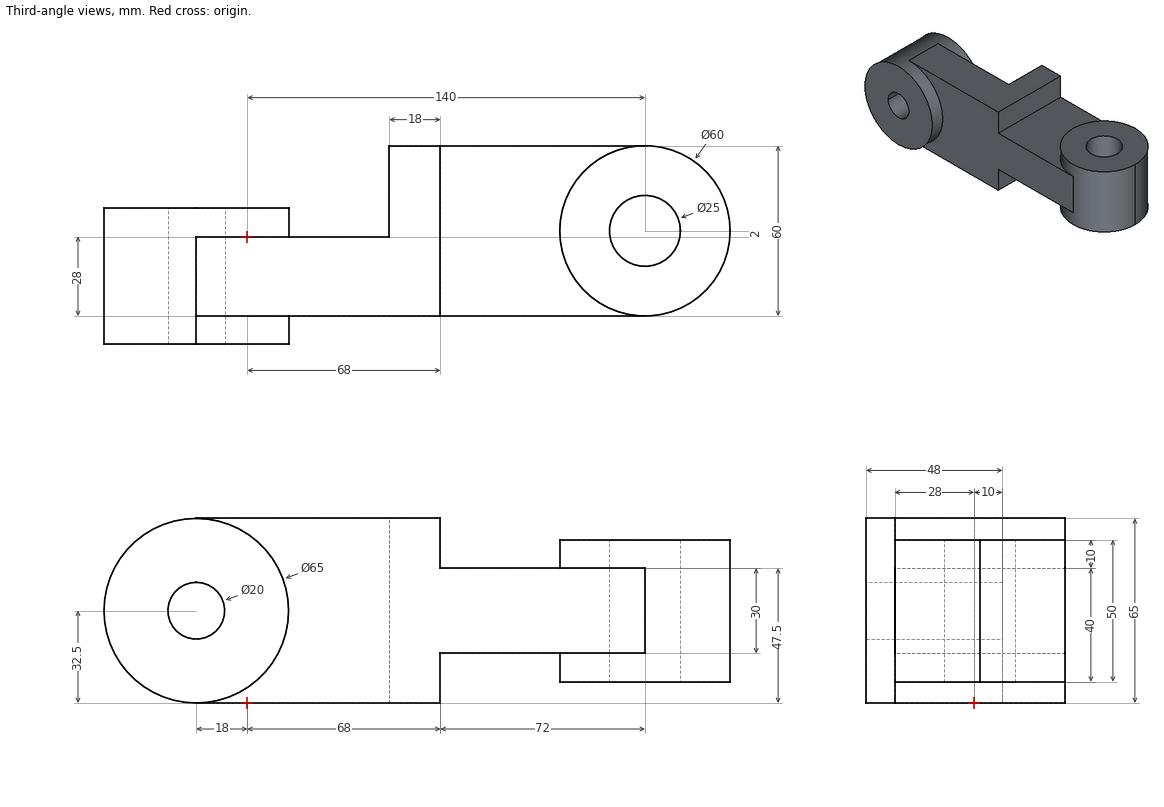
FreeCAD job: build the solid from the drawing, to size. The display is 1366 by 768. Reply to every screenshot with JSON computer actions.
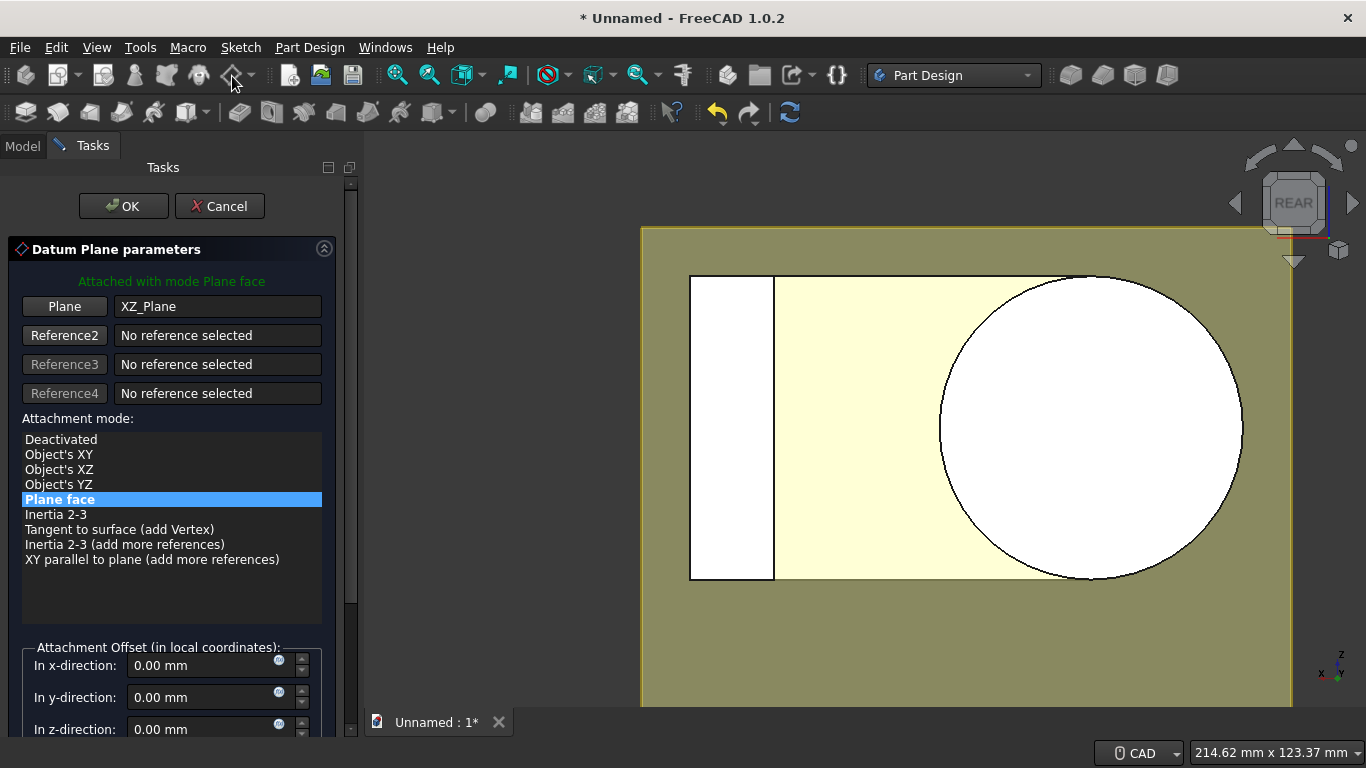
{"action": "scroll", "coordinate": [351, 456], "scroll_direction": "down", "scroll_amount": 2}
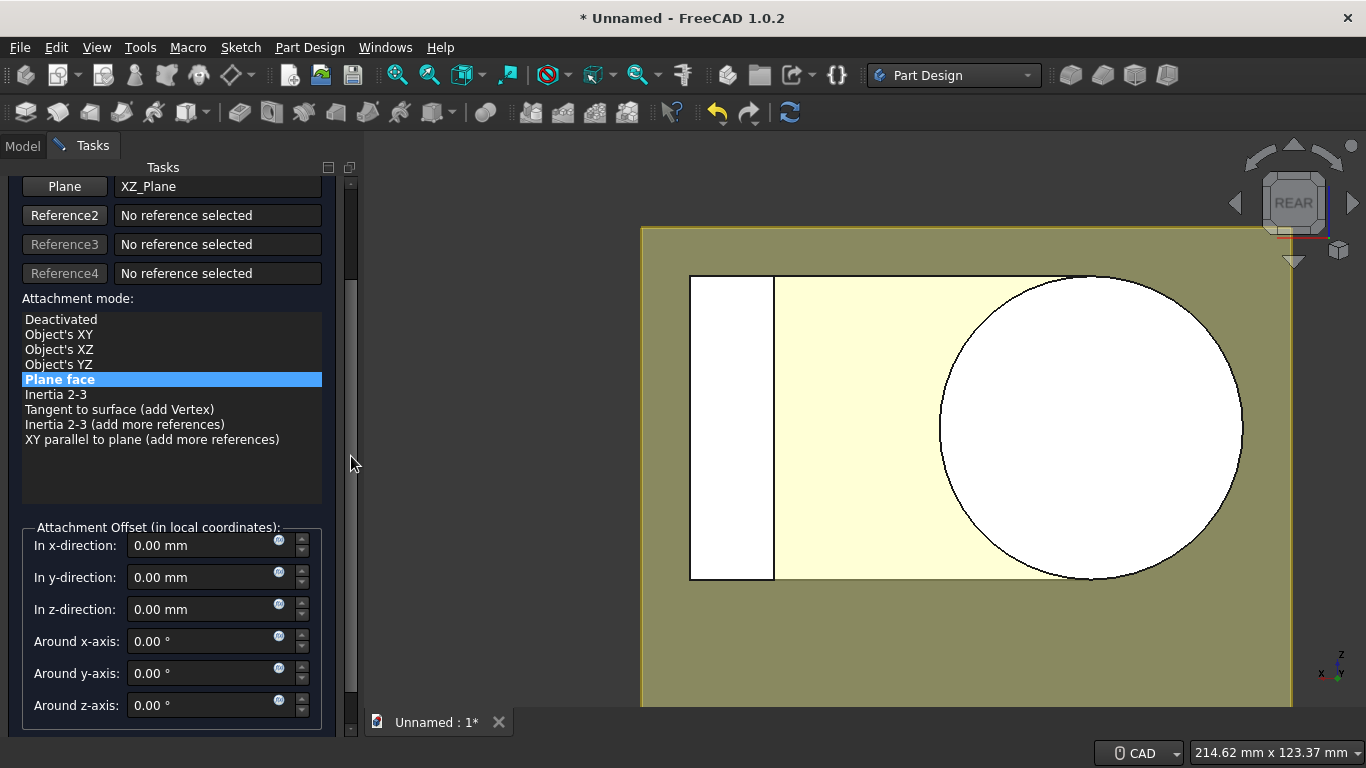
{"action": "triple_click", "coordinate": [210, 609]}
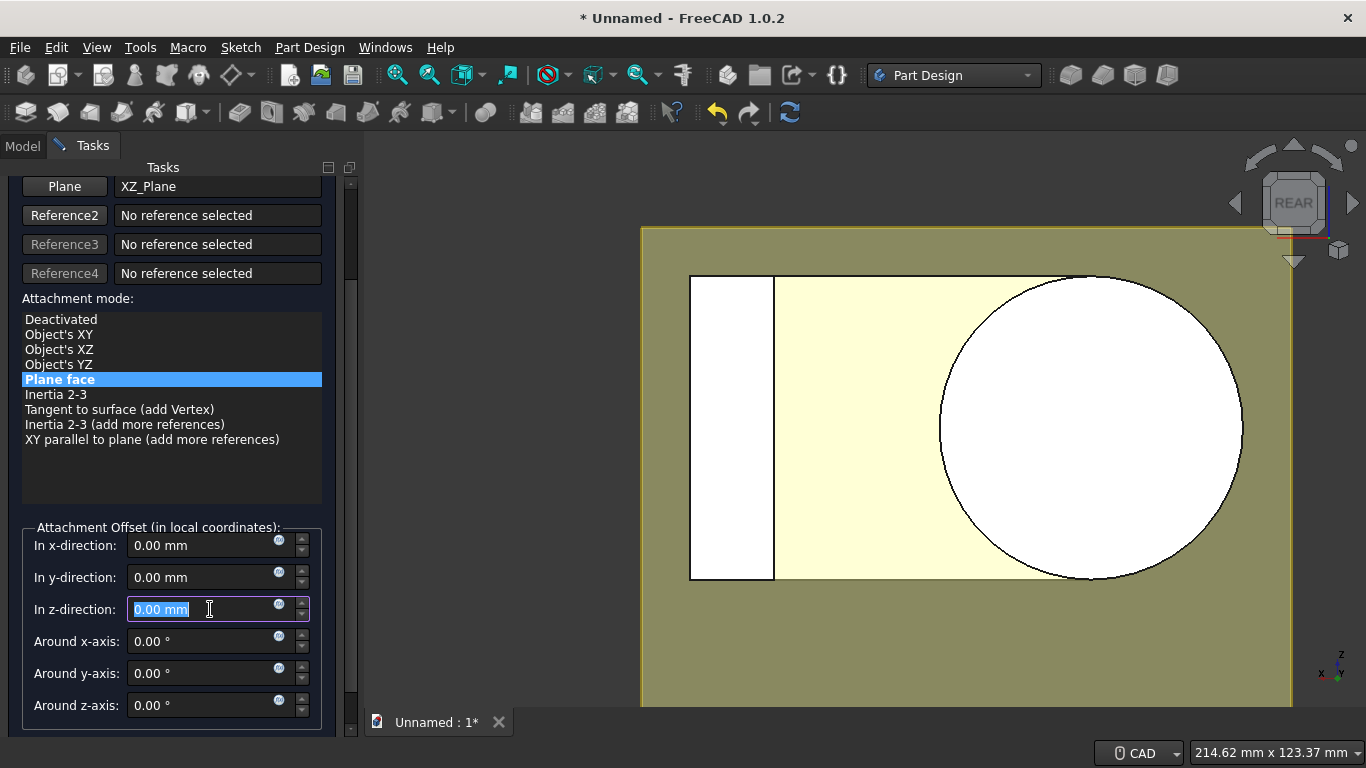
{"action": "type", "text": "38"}
{"action": "key", "text": "Tab"}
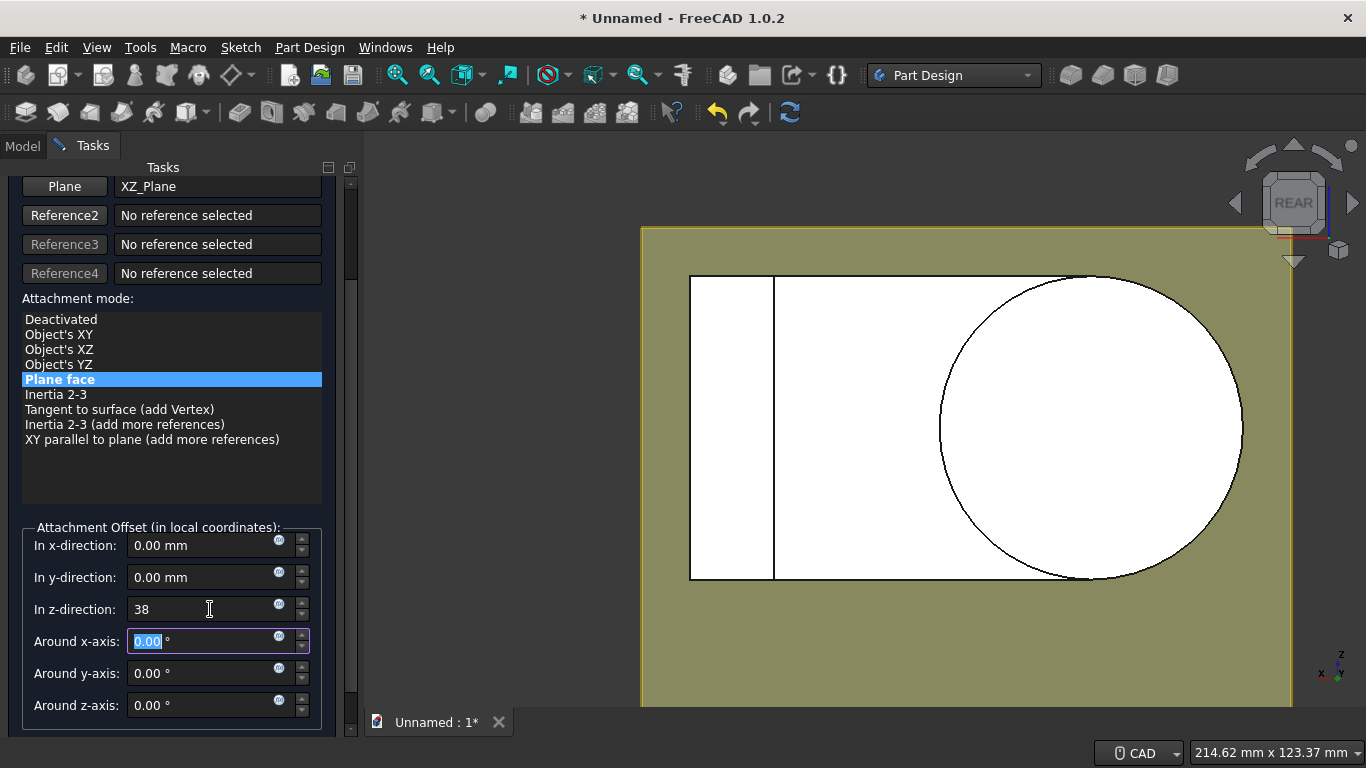
{"action": "scroll", "coordinate": [351, 456], "scroll_direction": "up", "scroll_amount": 3}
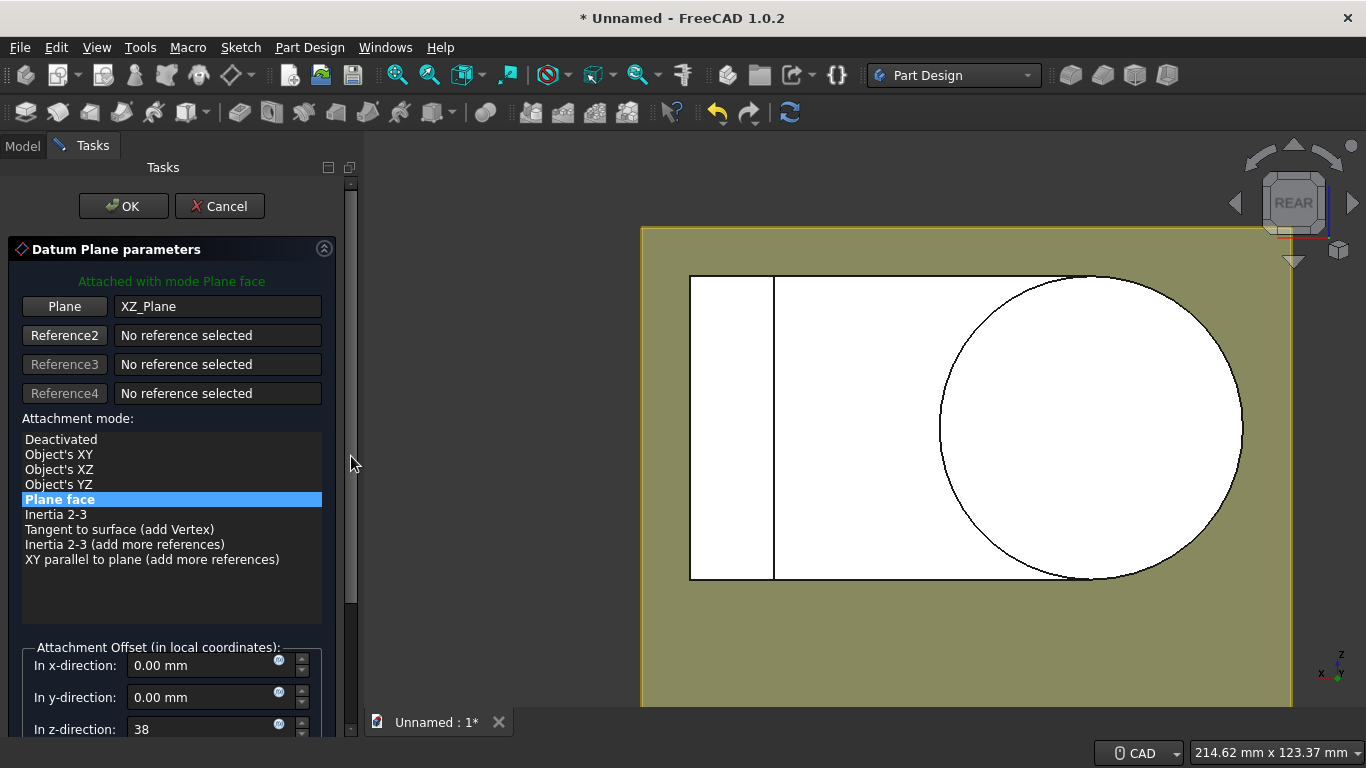
{"action": "left_click", "coordinate": [124, 206]}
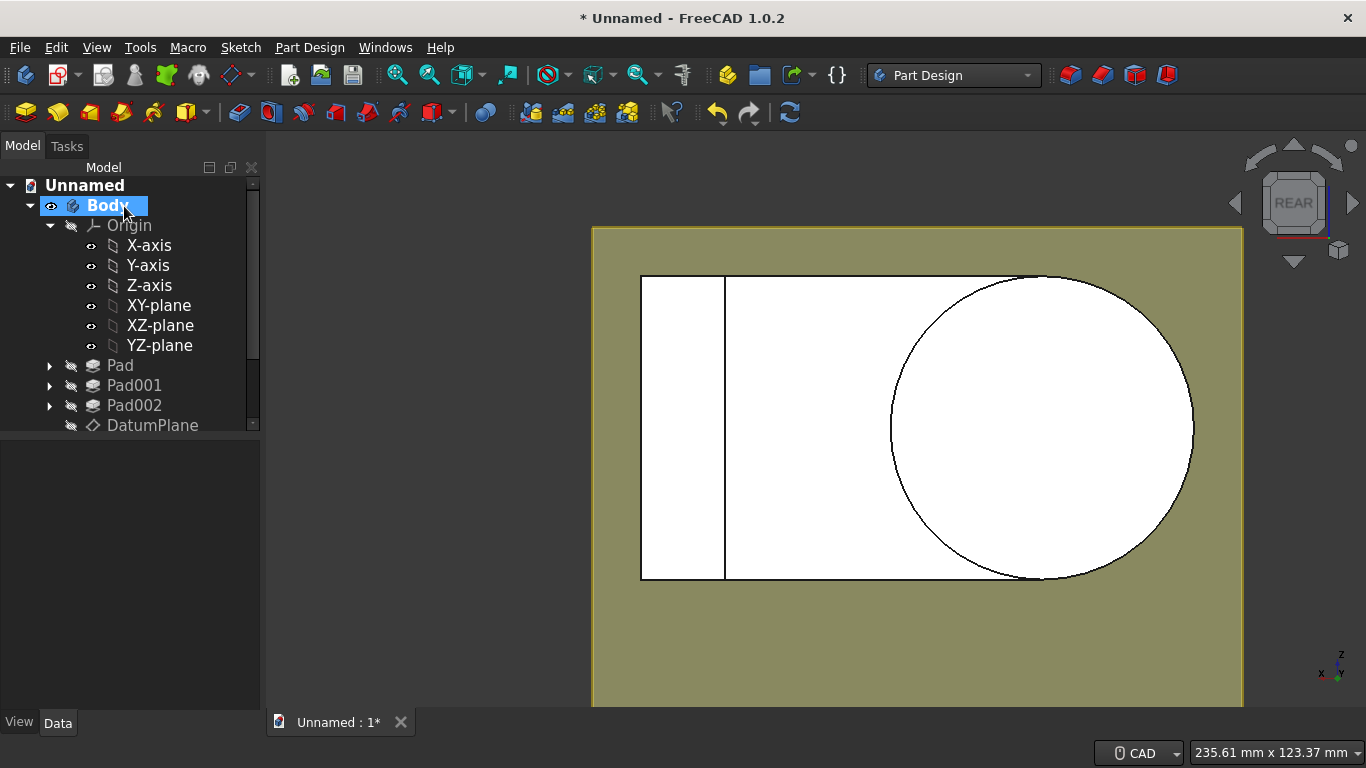
{"action": "scroll", "coordinate": [100, 301], "scroll_direction": "down", "scroll_amount": 3}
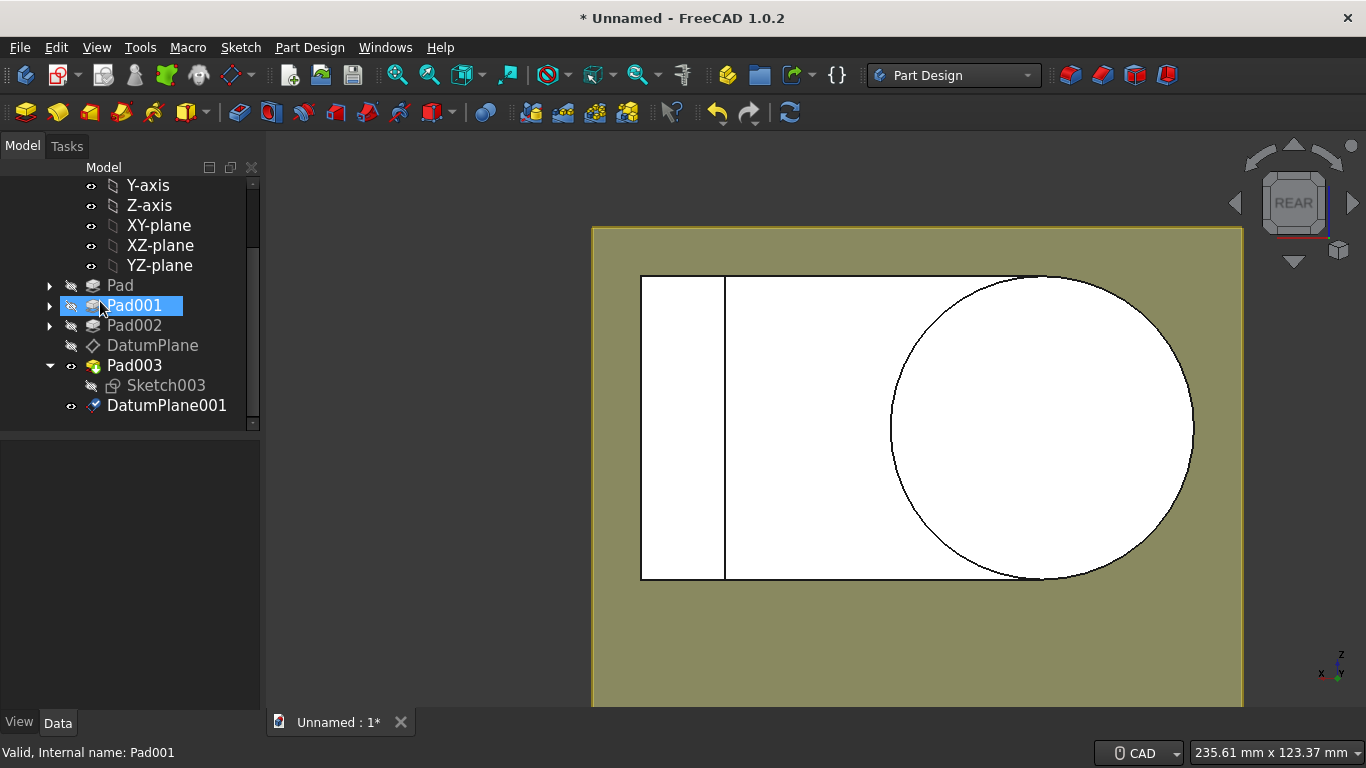
{"action": "left_click", "coordinate": [116, 406]}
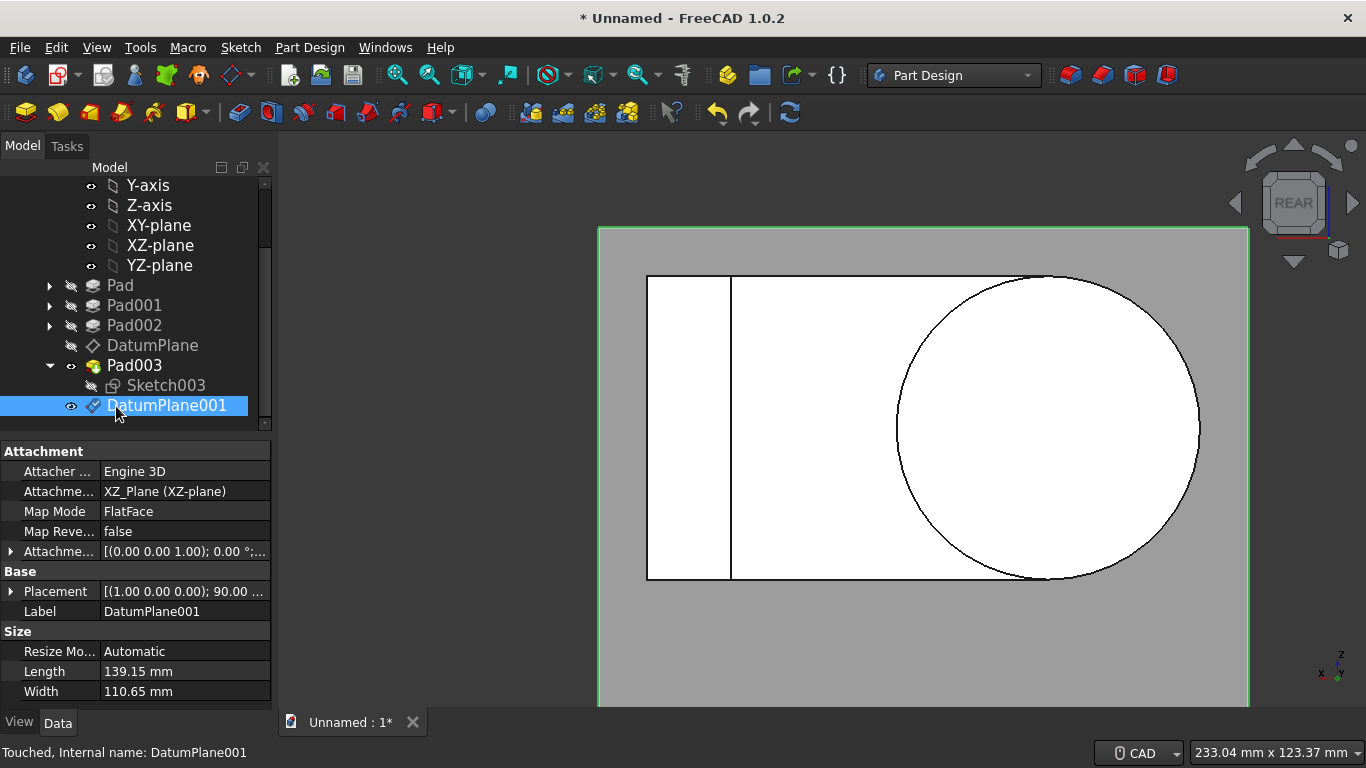
{"action": "left_click", "coordinate": [58, 76]}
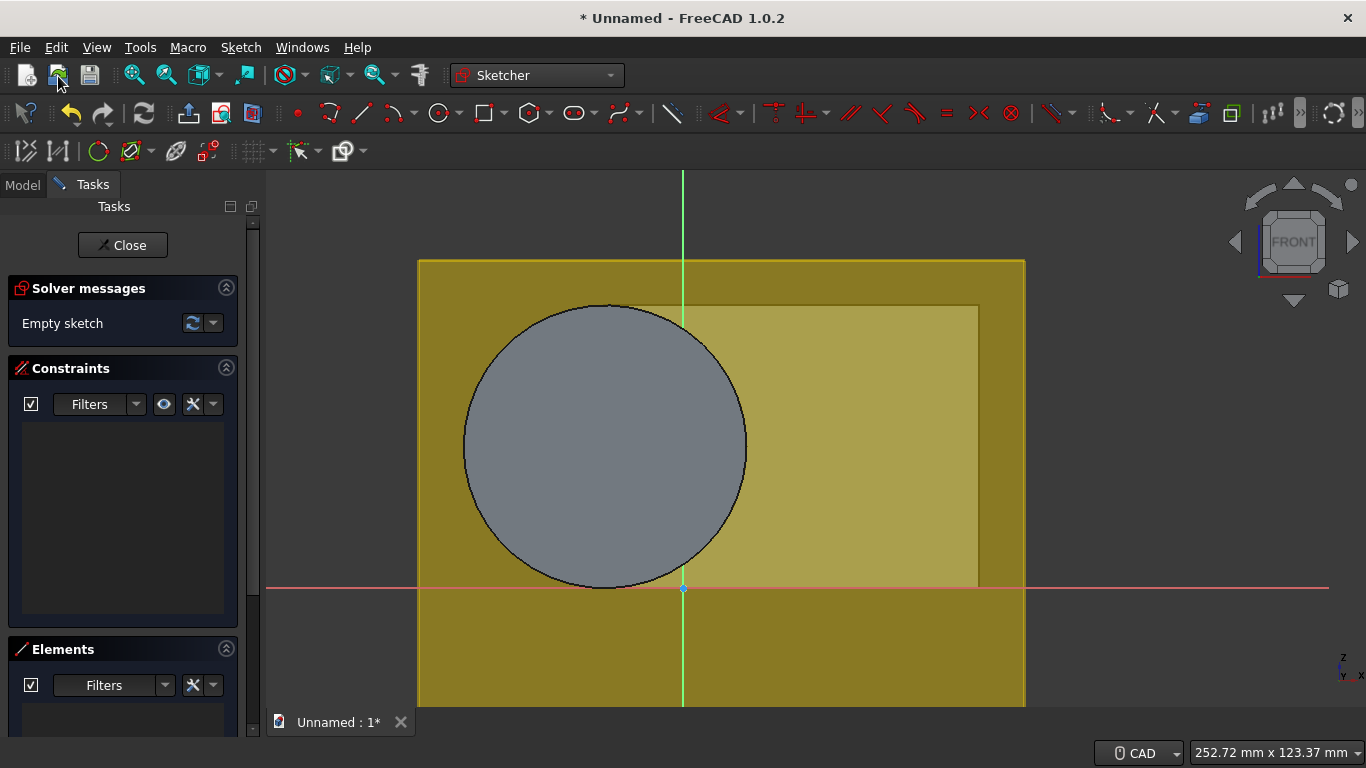
{"action": "key", "text": "q s"}